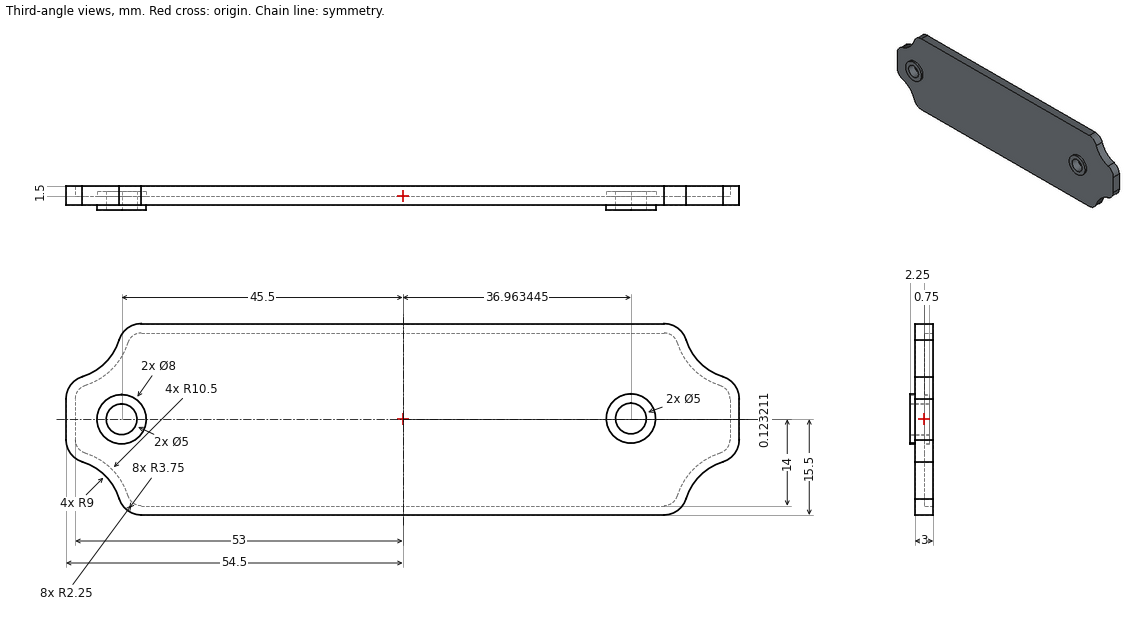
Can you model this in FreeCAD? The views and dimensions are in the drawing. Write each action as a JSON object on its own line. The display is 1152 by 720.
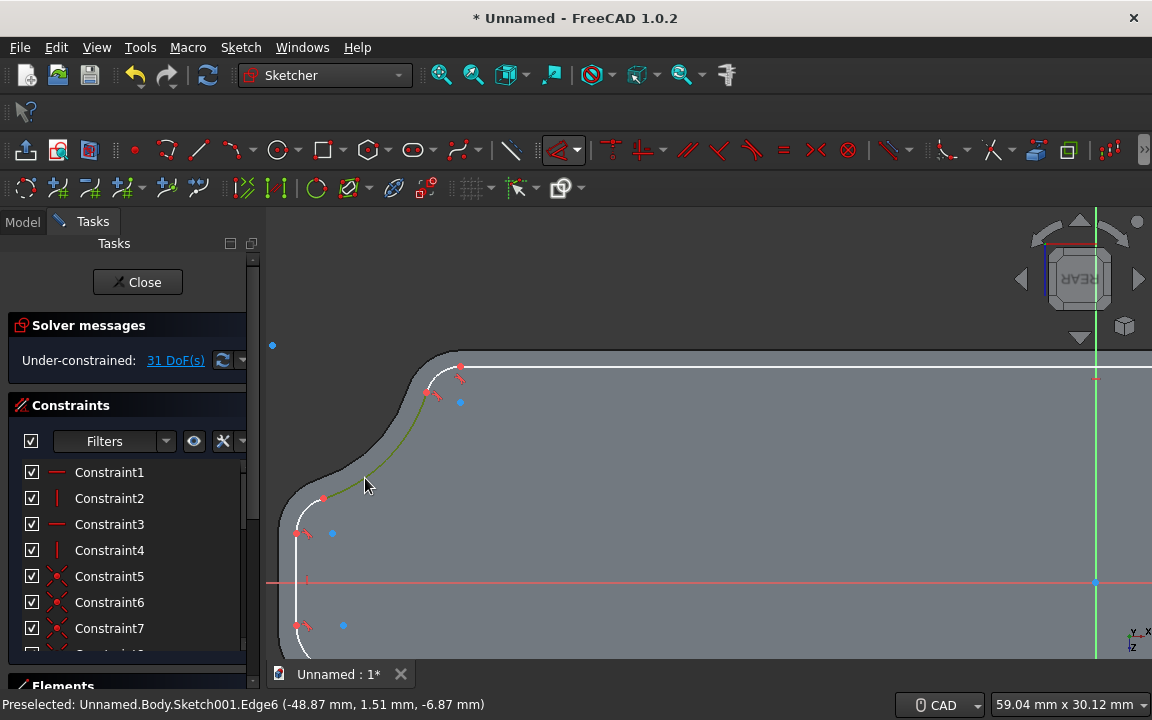
{"action": "left_click", "coordinate": [311, 505]}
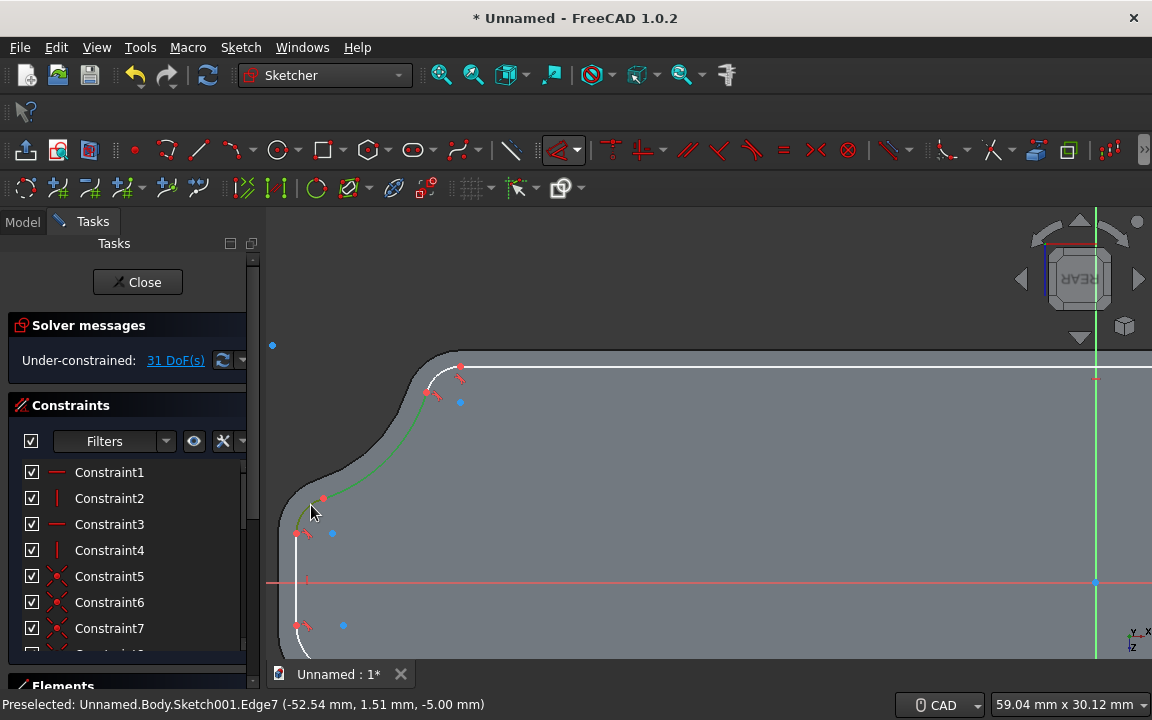
{"action": "left_click", "coordinate": [752, 150]}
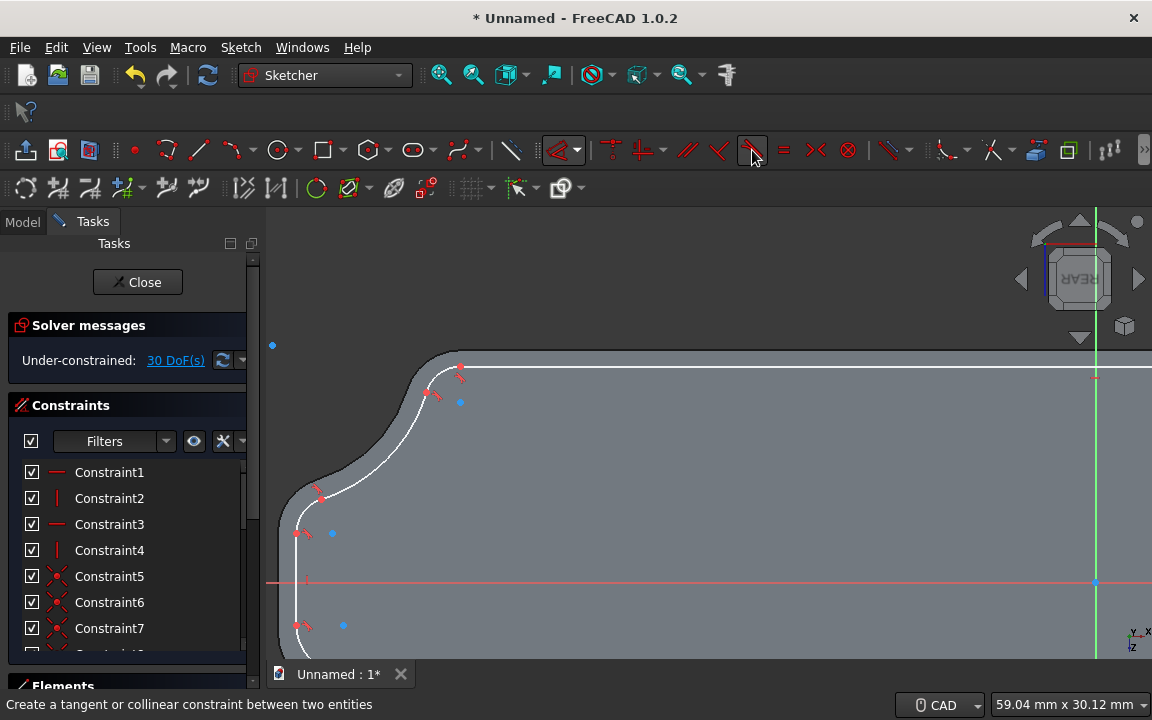
{"action": "scroll", "coordinate": [444, 368], "scroll_direction": "down", "scroll_amount": 6}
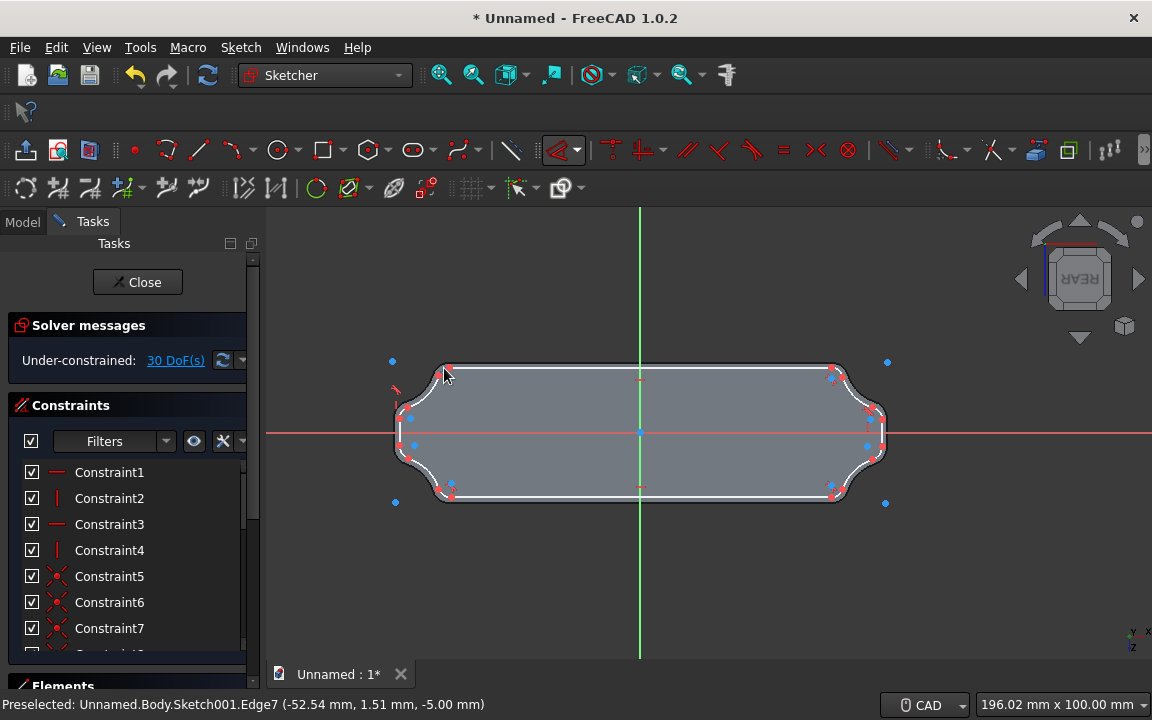
{"action": "scroll", "coordinate": [401, 450], "scroll_direction": "up", "scroll_amount": 6}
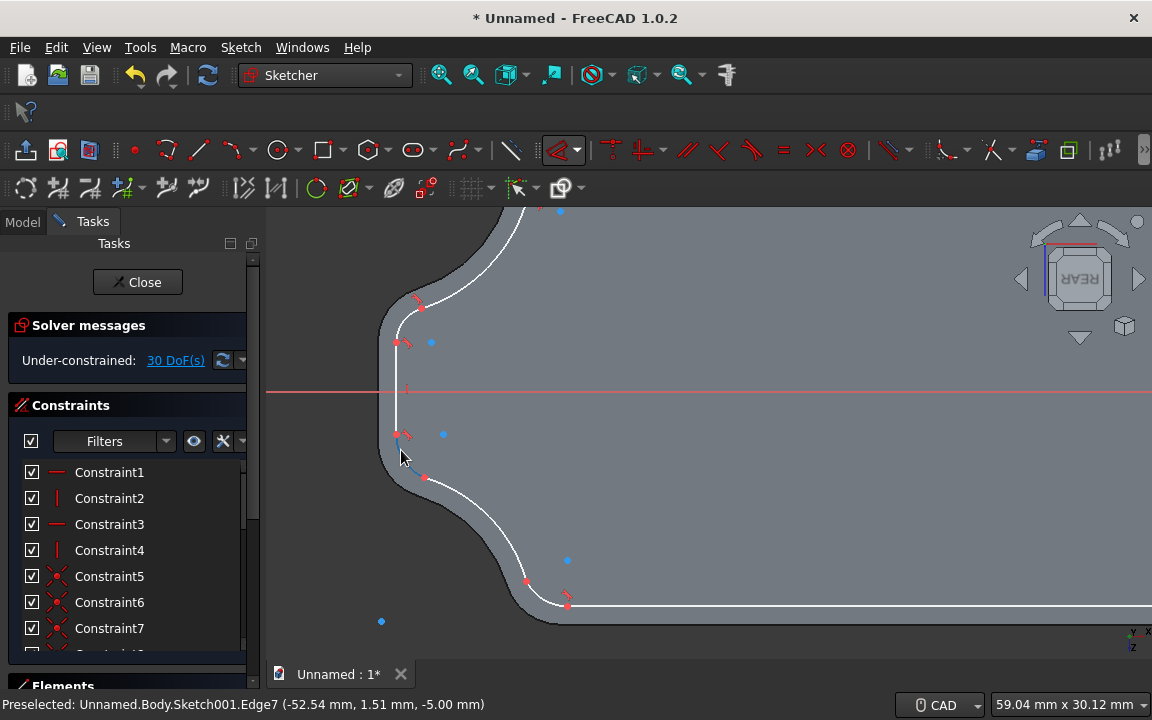
{"action": "left_click", "coordinate": [399, 450]}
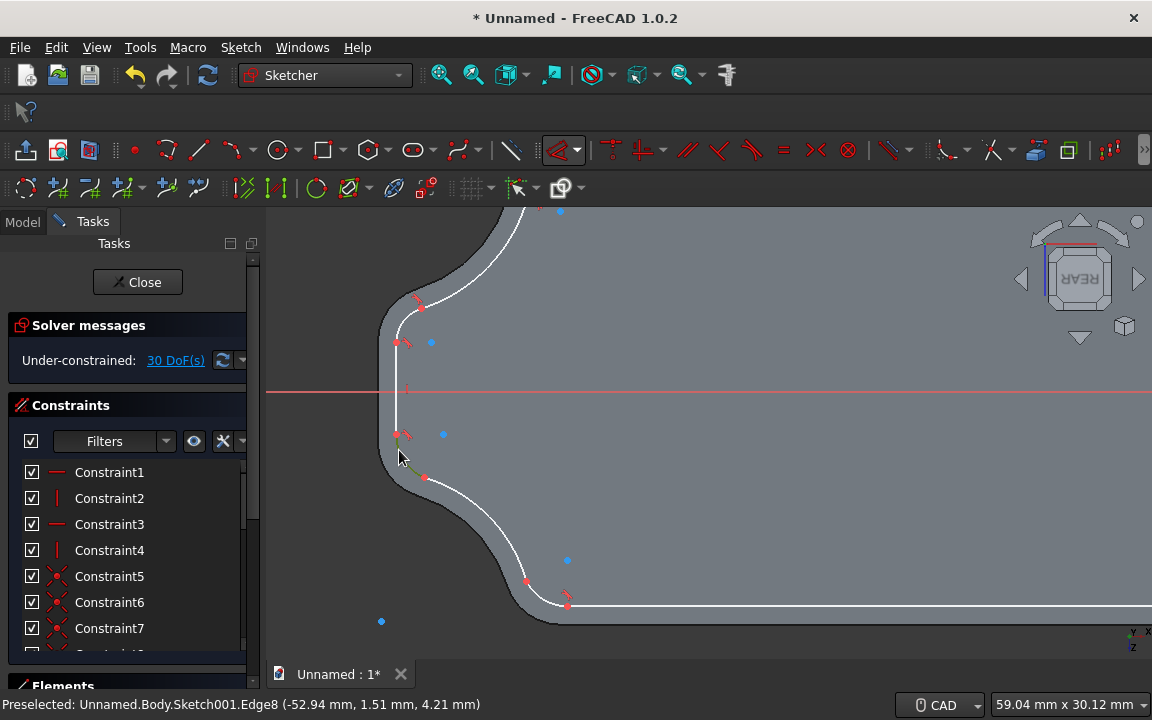
{"action": "left_click", "coordinate": [508, 540]}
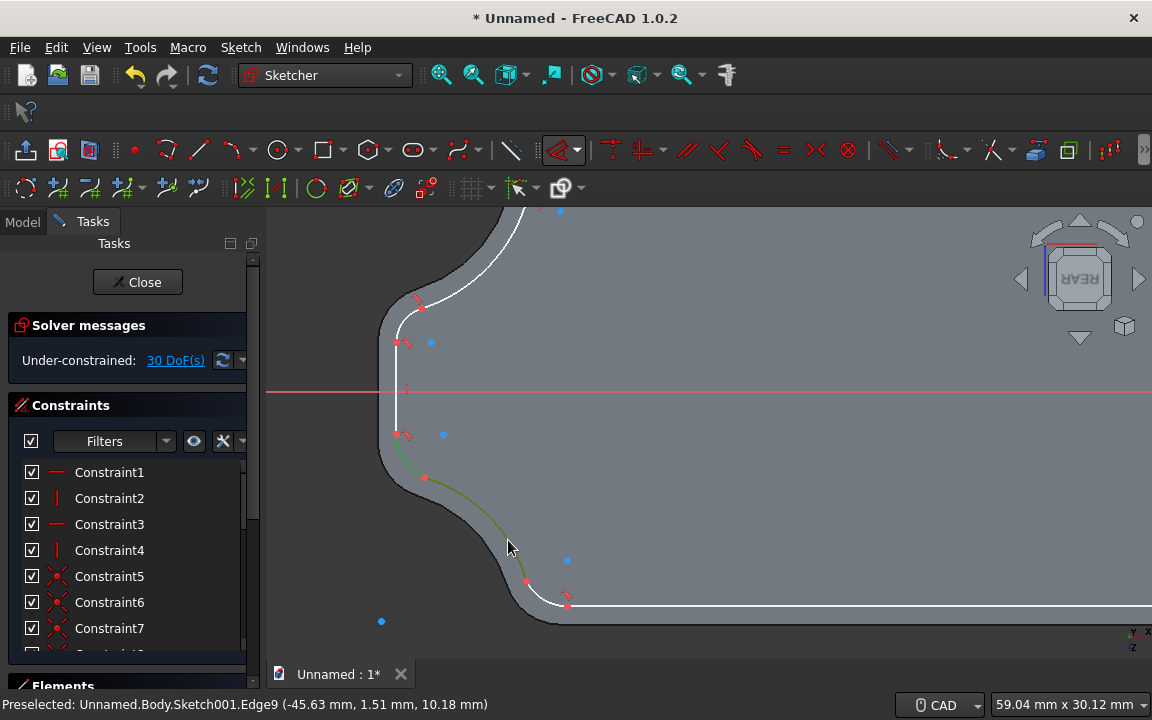
{"action": "left_click", "coordinate": [752, 150]}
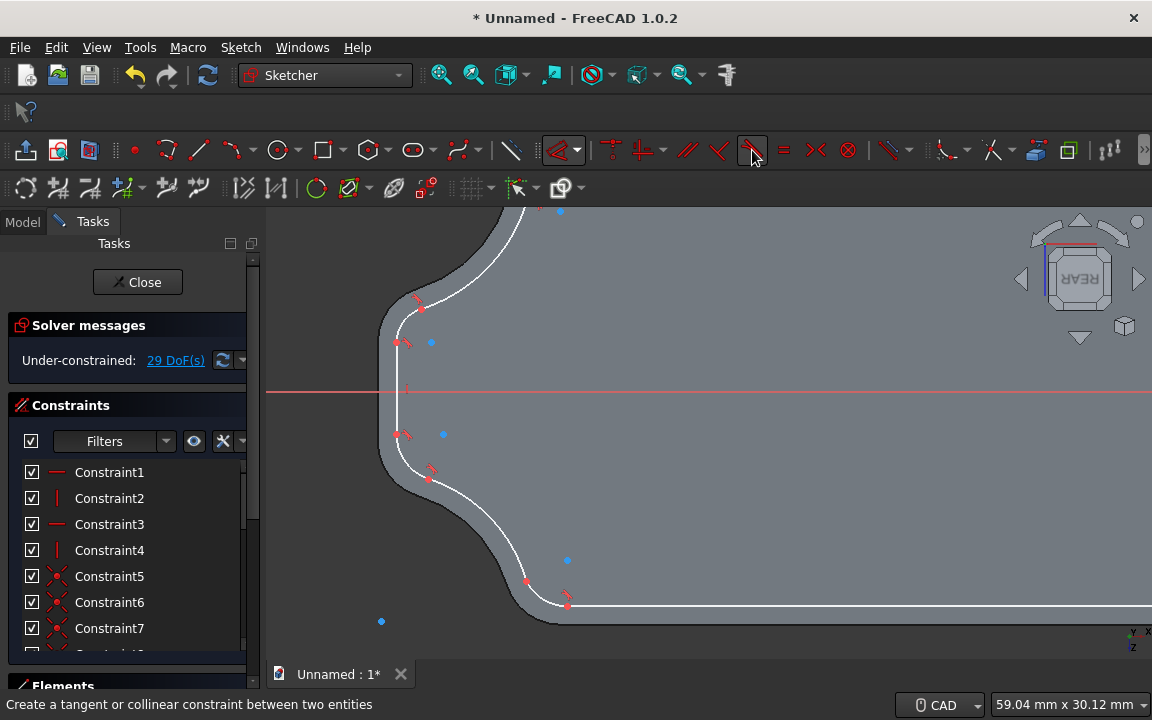
{"action": "left_click", "coordinate": [509, 541]}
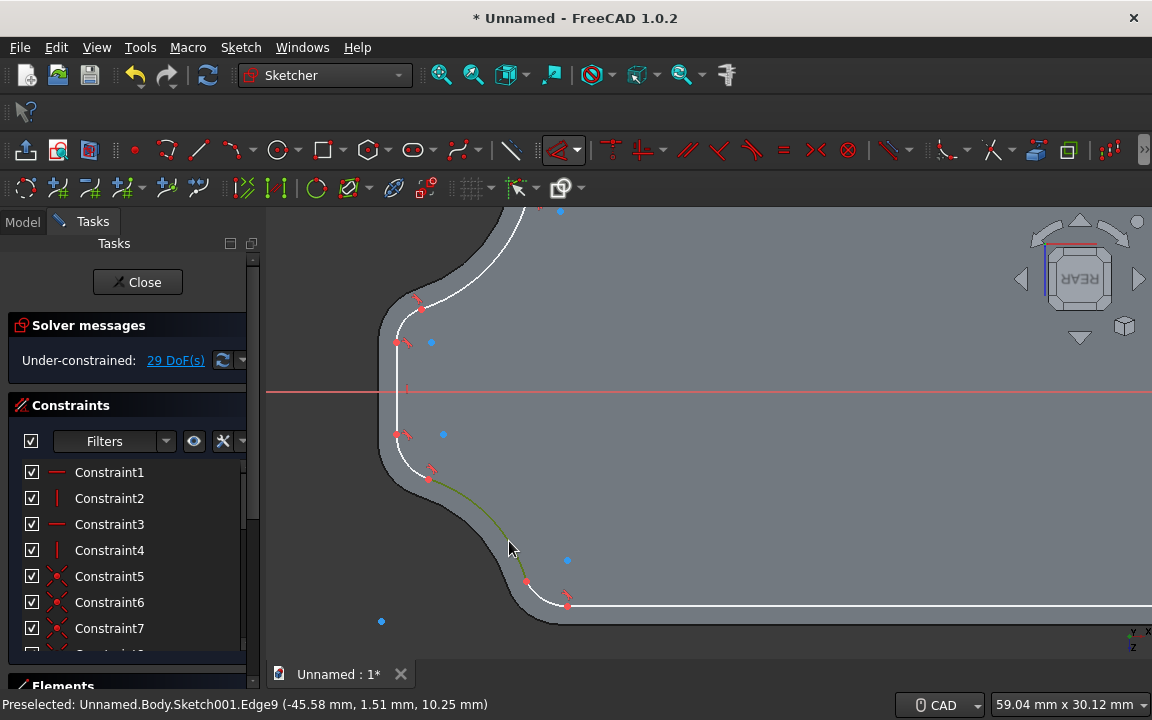
{"action": "left_click", "coordinate": [535, 593]}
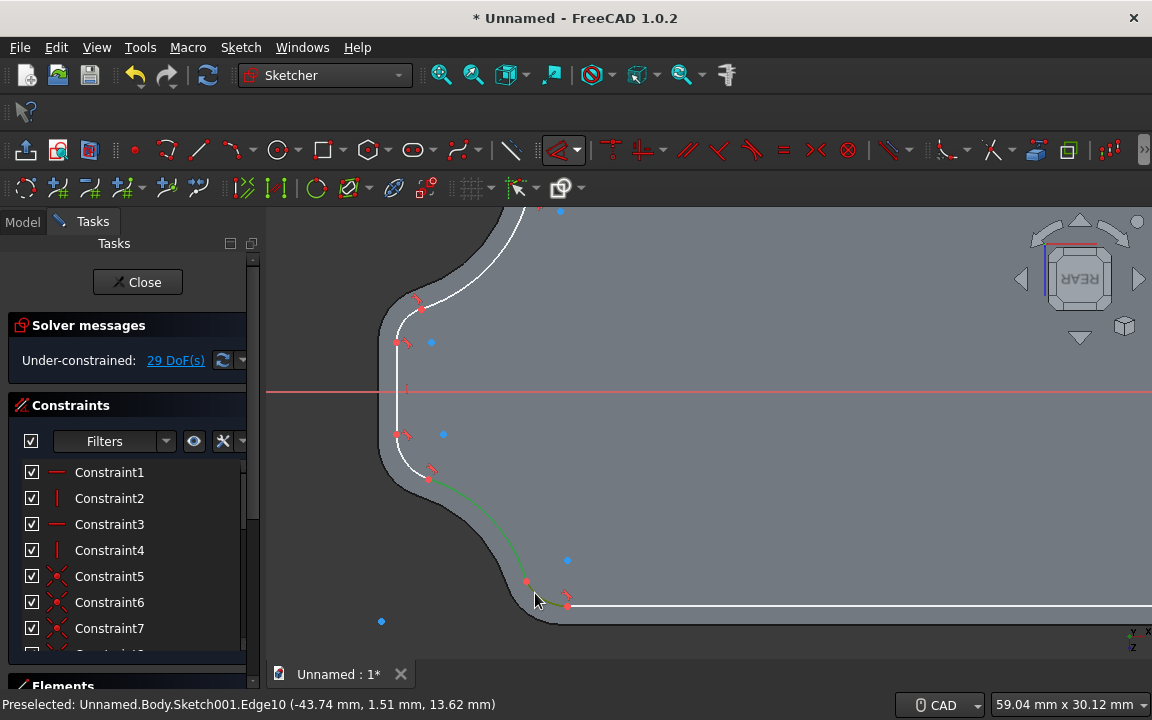
{"action": "left_click", "coordinate": [752, 150]}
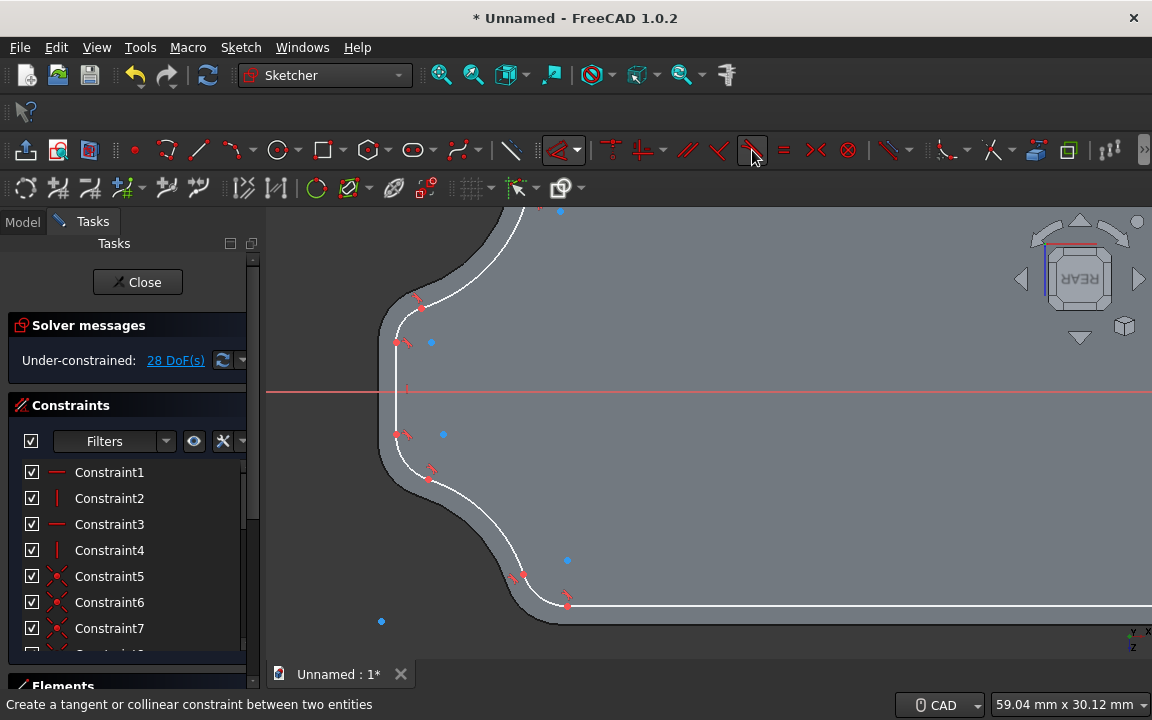
{"action": "scroll", "coordinate": [401, 451], "scroll_direction": "down", "scroll_amount": 6}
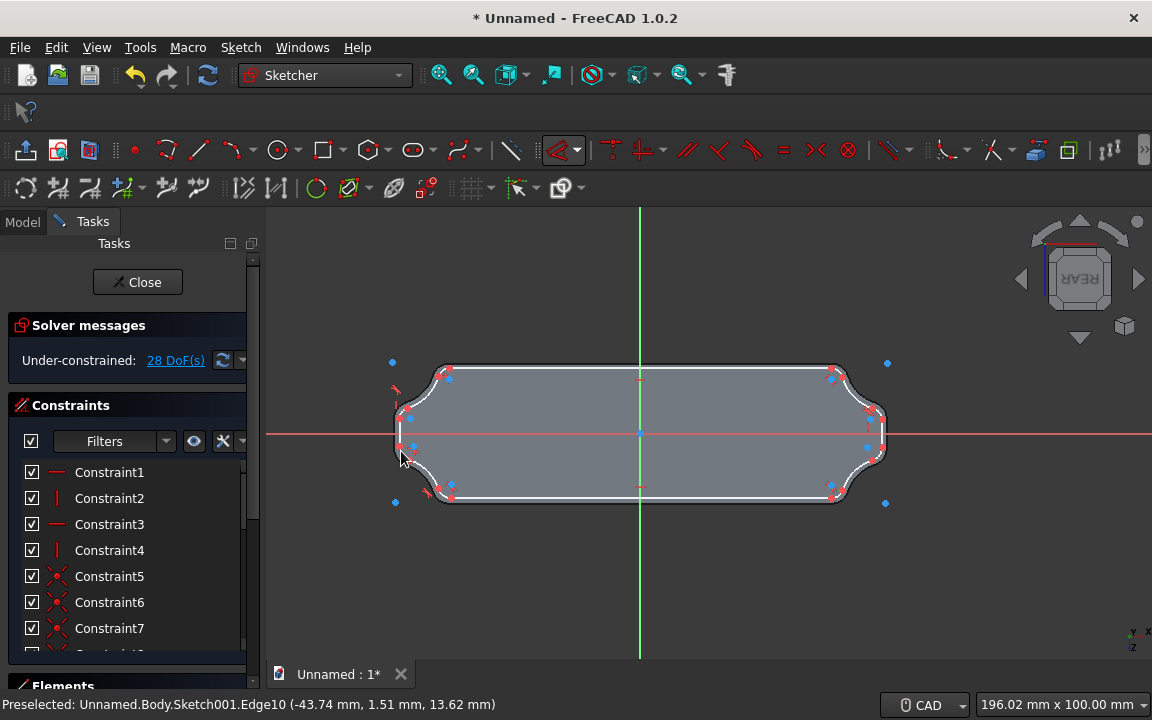
{"action": "scroll", "coordinate": [836, 497], "scroll_direction": "up", "scroll_amount": 6}